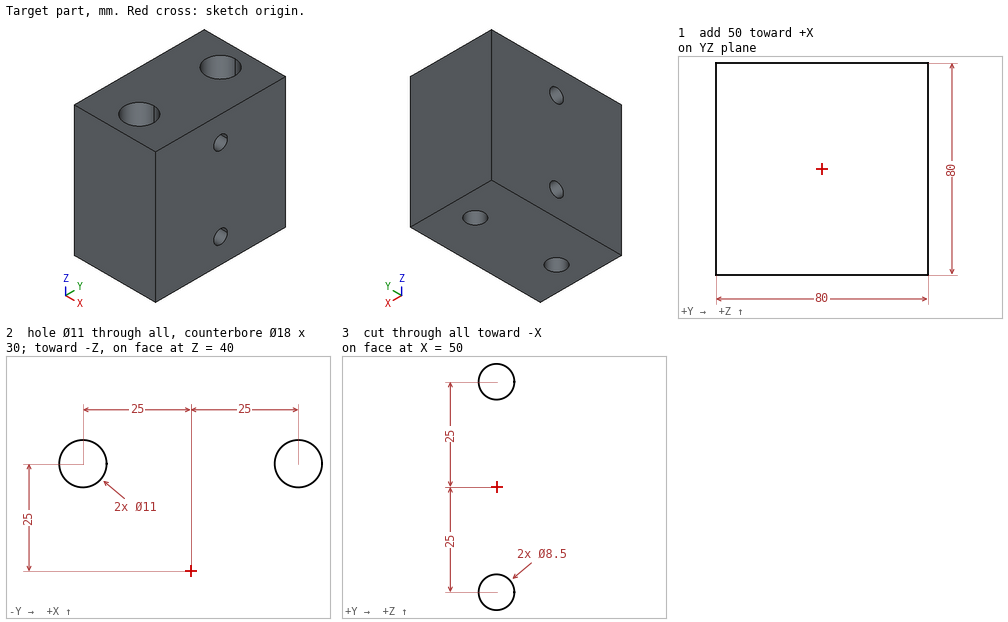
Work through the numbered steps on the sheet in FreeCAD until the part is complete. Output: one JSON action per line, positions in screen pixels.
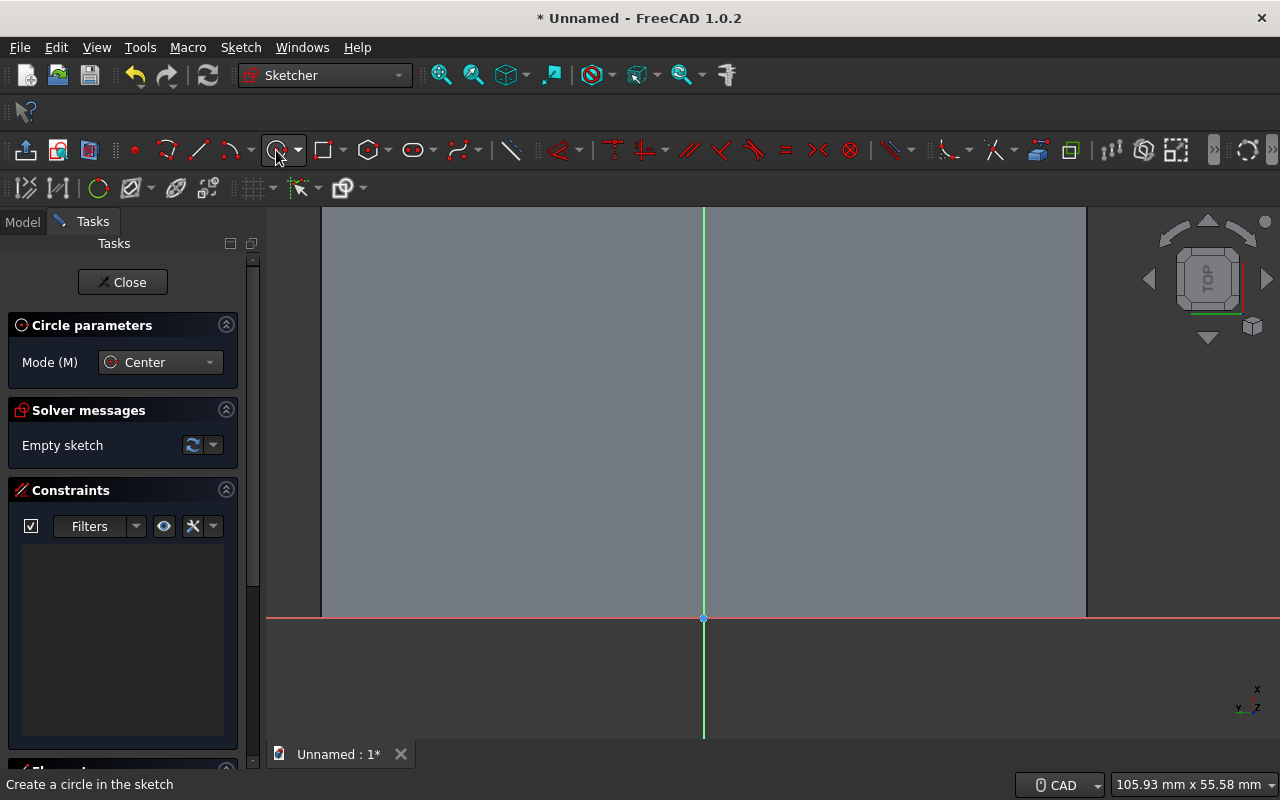
{"action": "left_click", "coordinate": [464, 379]}
{"action": "left_click", "coordinate": [502, 342]}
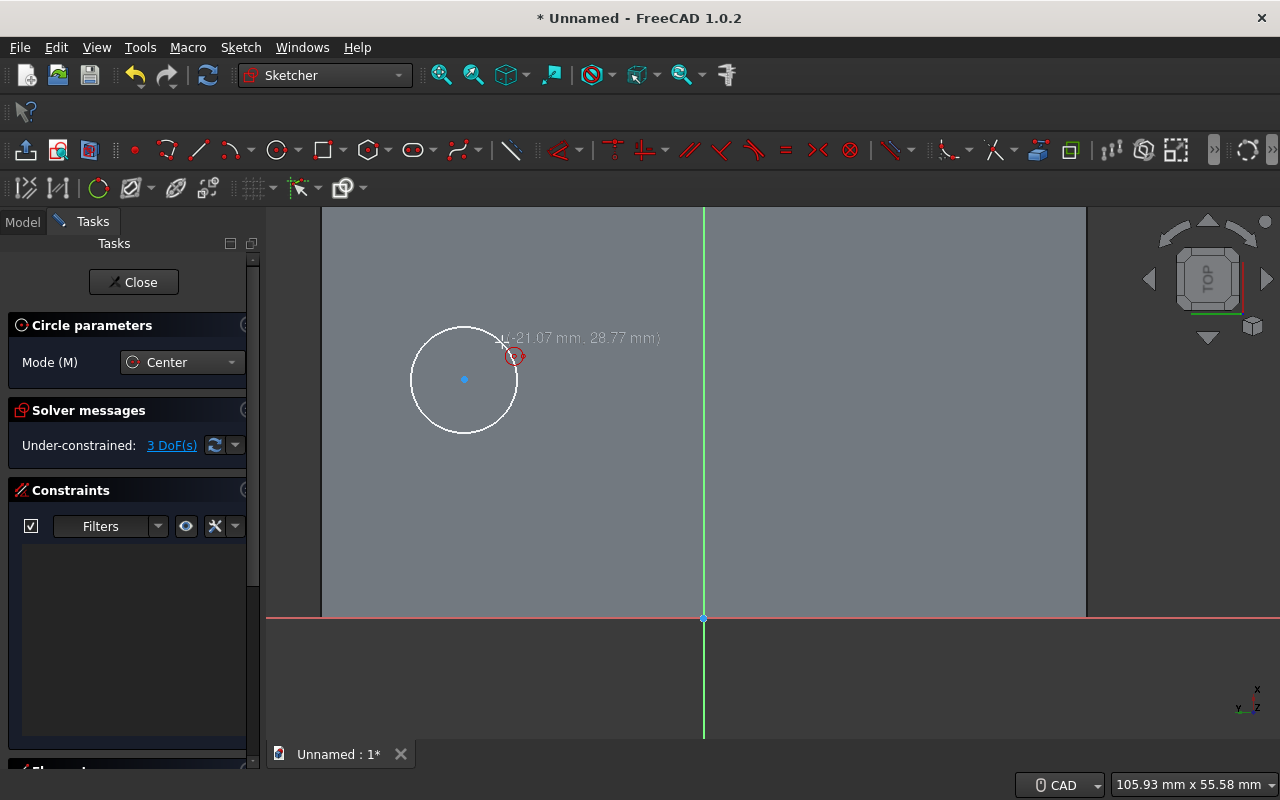
{"action": "left_click", "coordinate": [943, 379]}
{"action": "left_click", "coordinate": [980, 342]}
{"action": "key", "text": "Escape"}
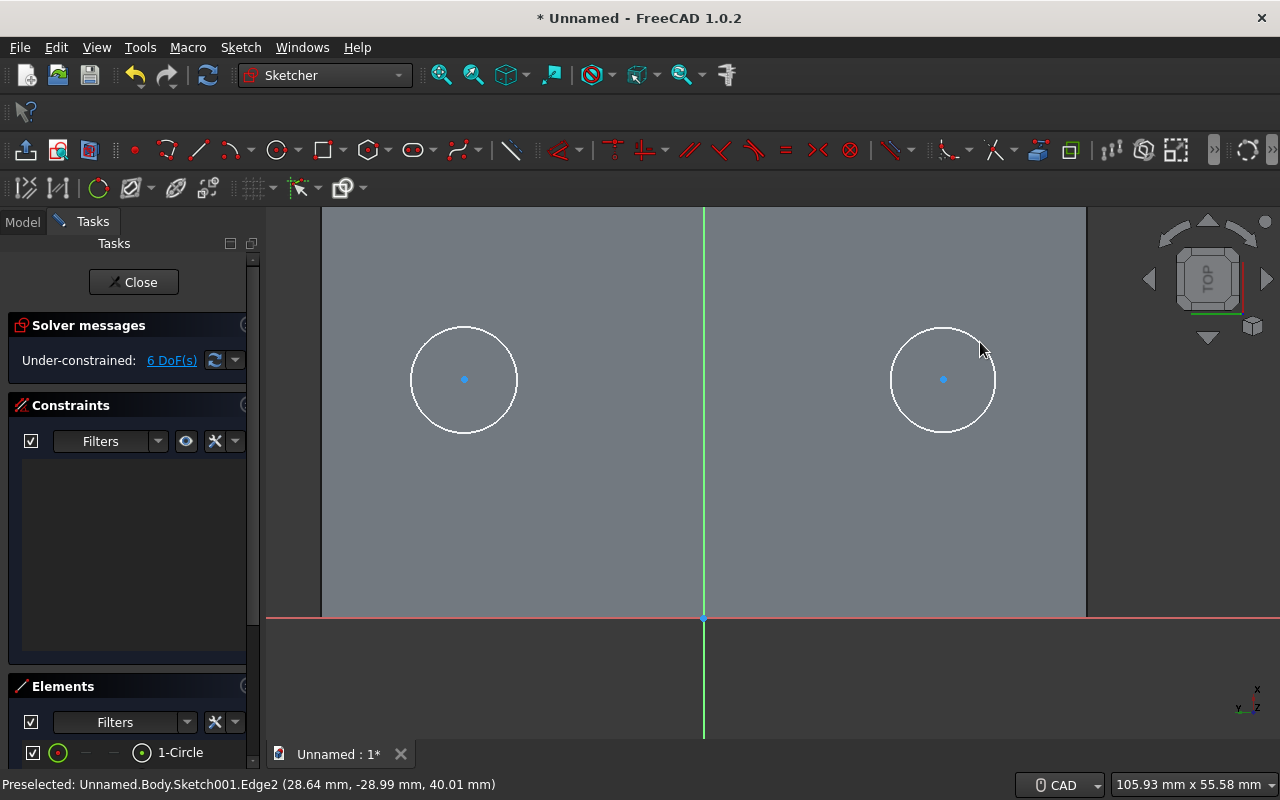
{"action": "left_click", "coordinate": [501, 342]}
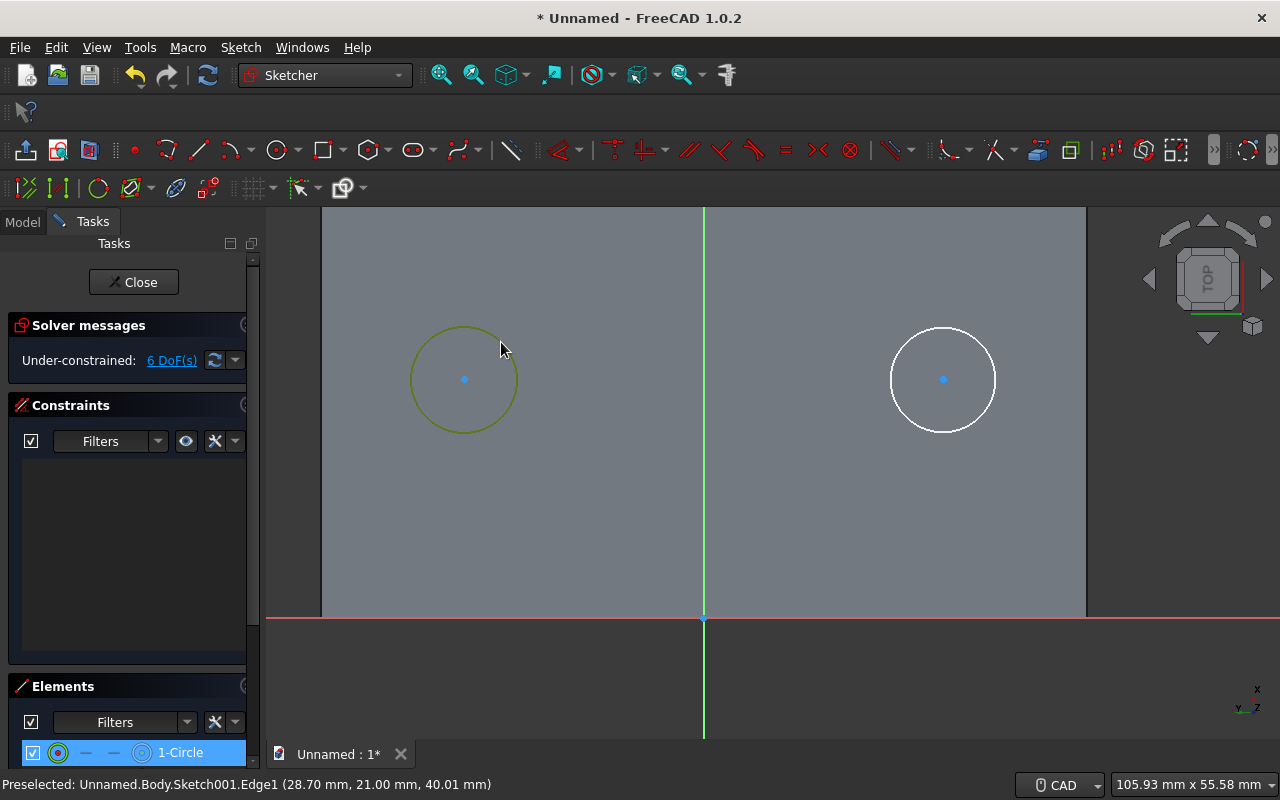
{"action": "left_click", "coordinate": [980, 343]}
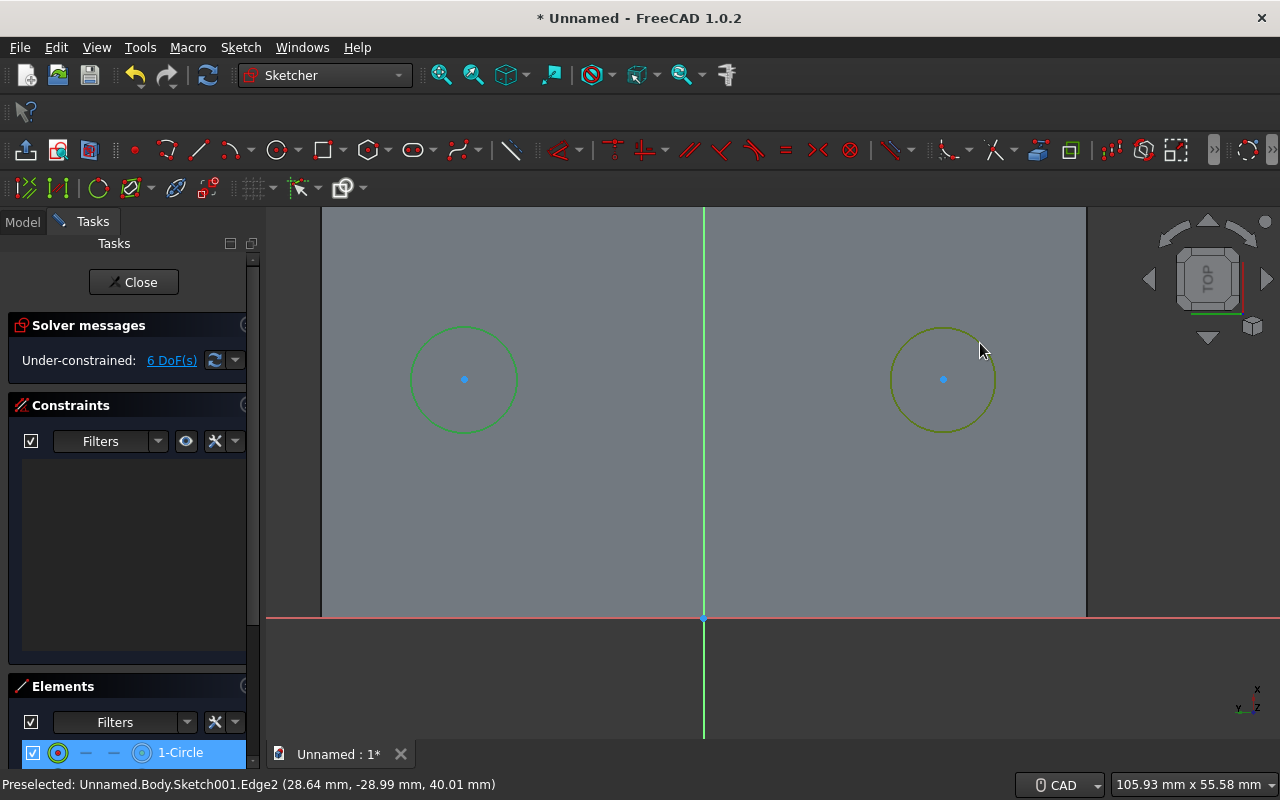
{"action": "left_click", "coordinate": [786, 150]}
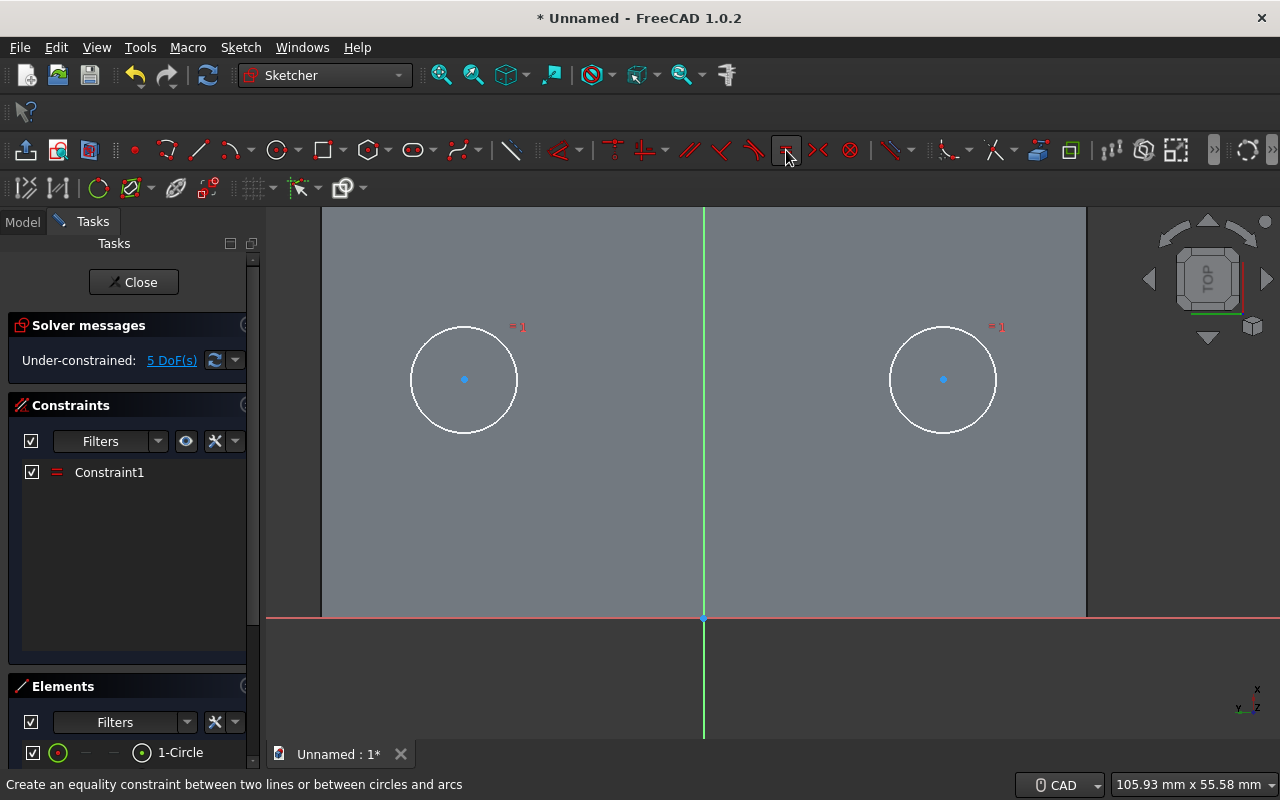
{"action": "left_click", "coordinate": [464, 380]}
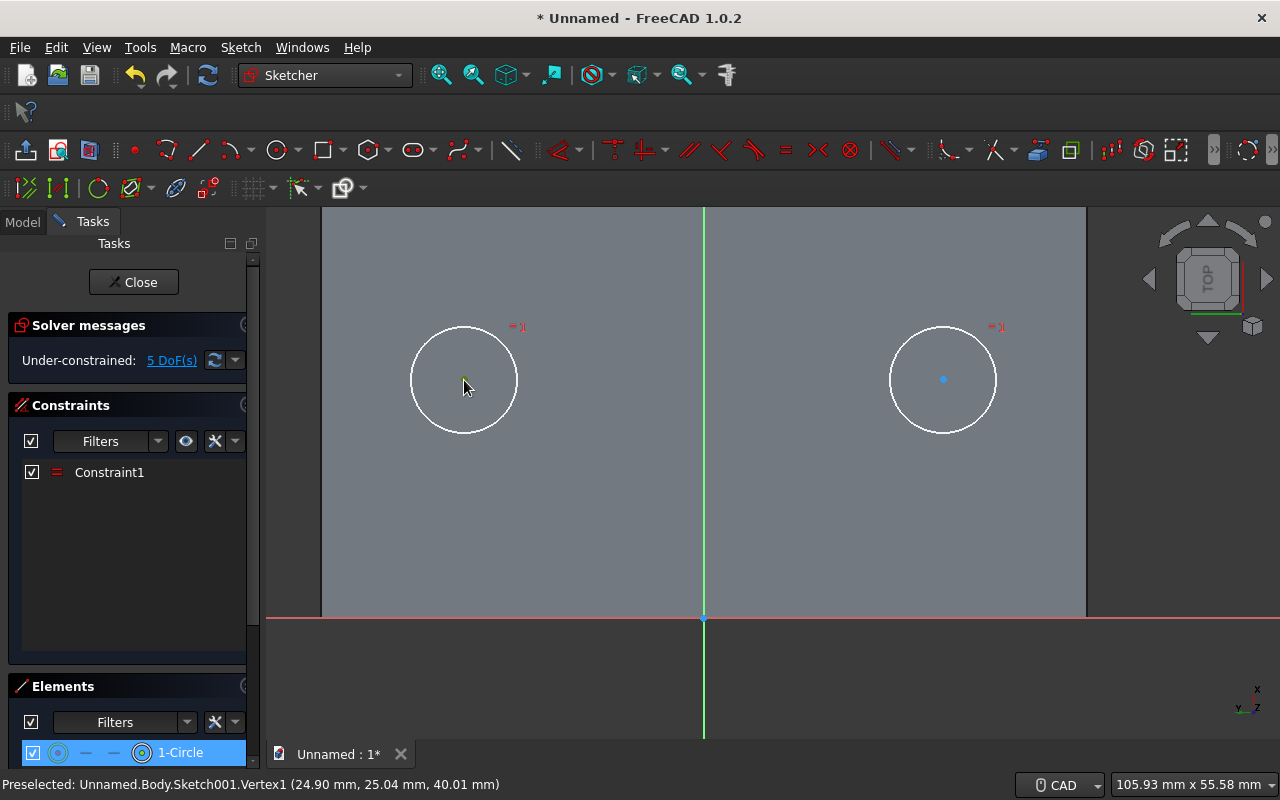
{"action": "left_click", "coordinate": [943, 380]}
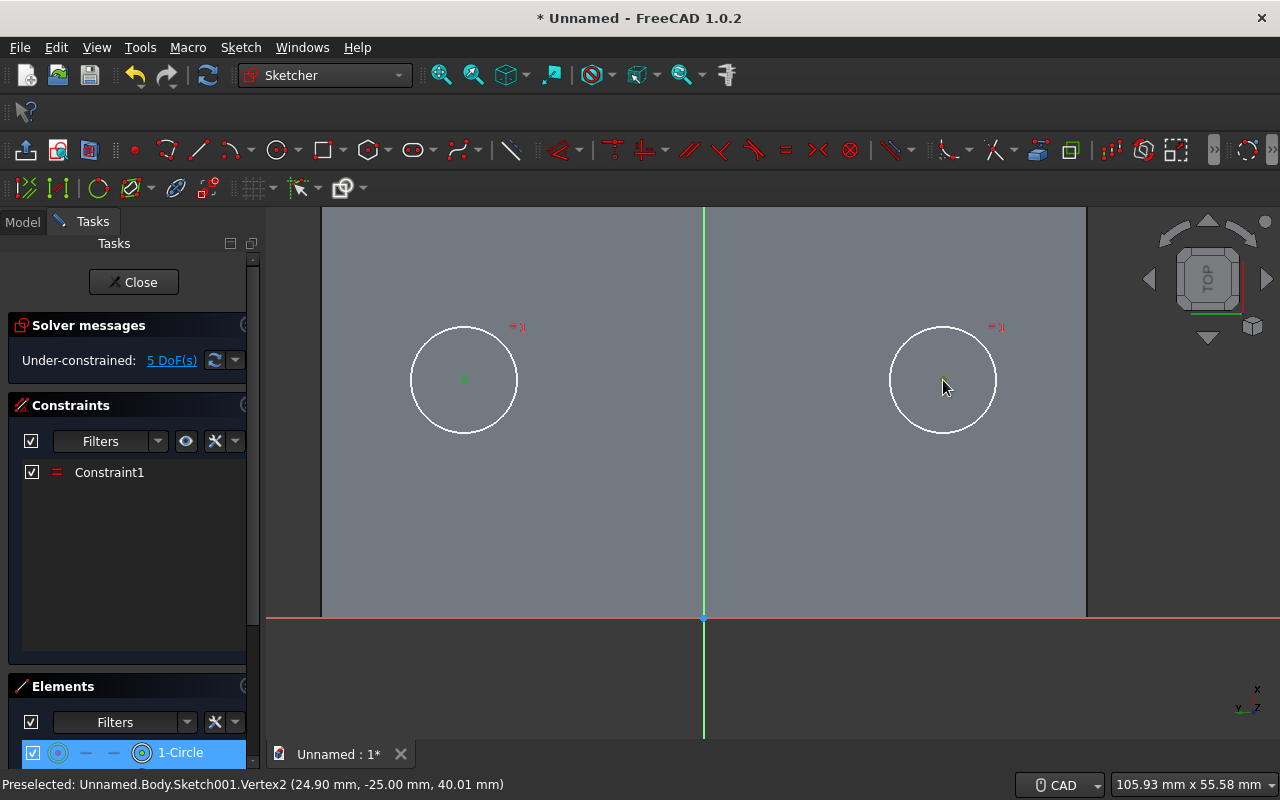
{"action": "key", "text": "h"}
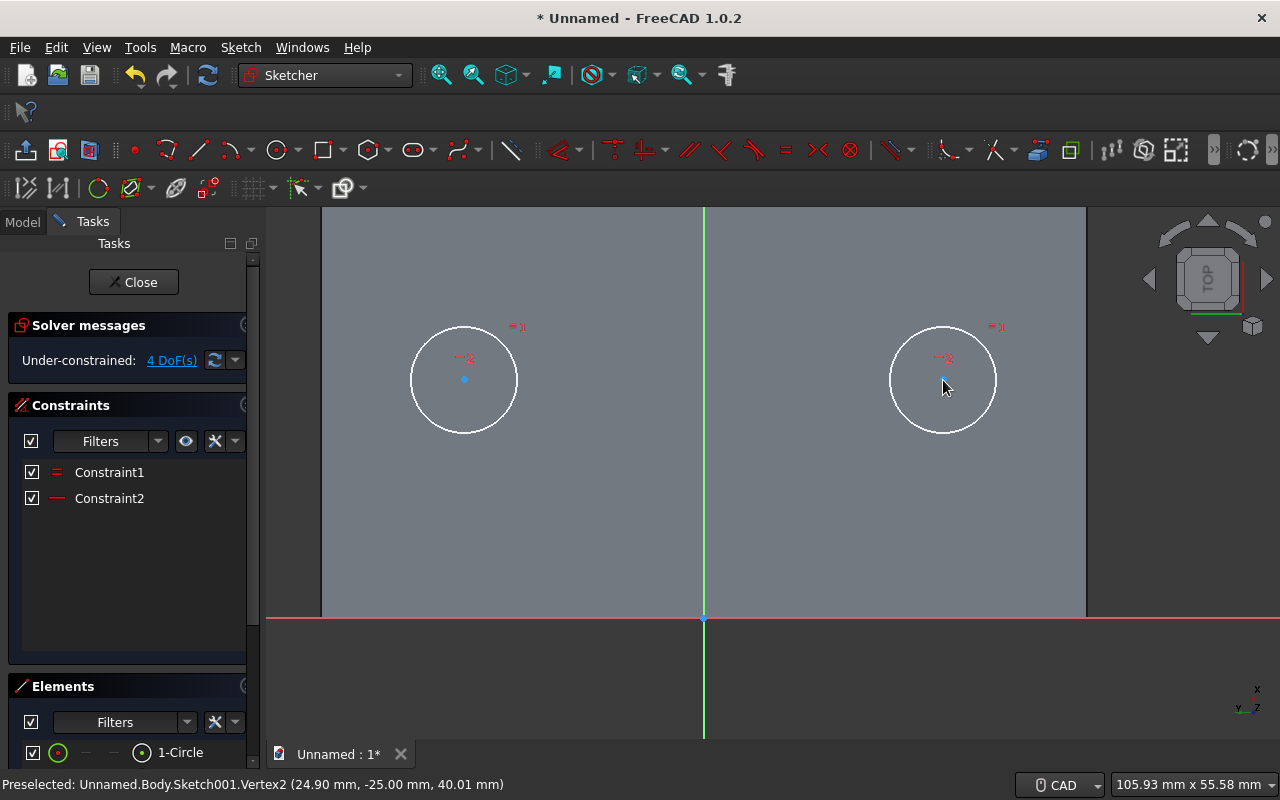
{"action": "left_click", "coordinate": [558, 150]}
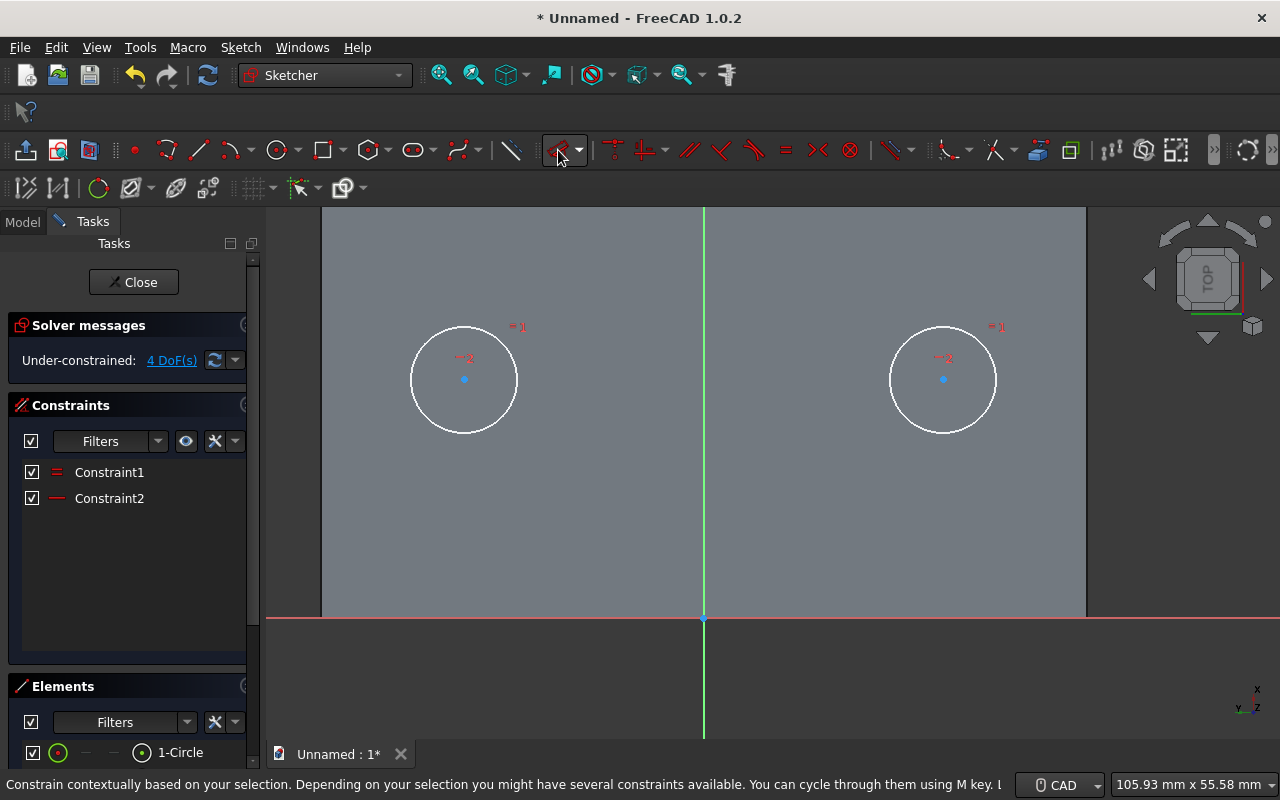
{"action": "left_click", "coordinate": [501, 342]}
{"action": "left_click", "coordinate": [523, 319]}